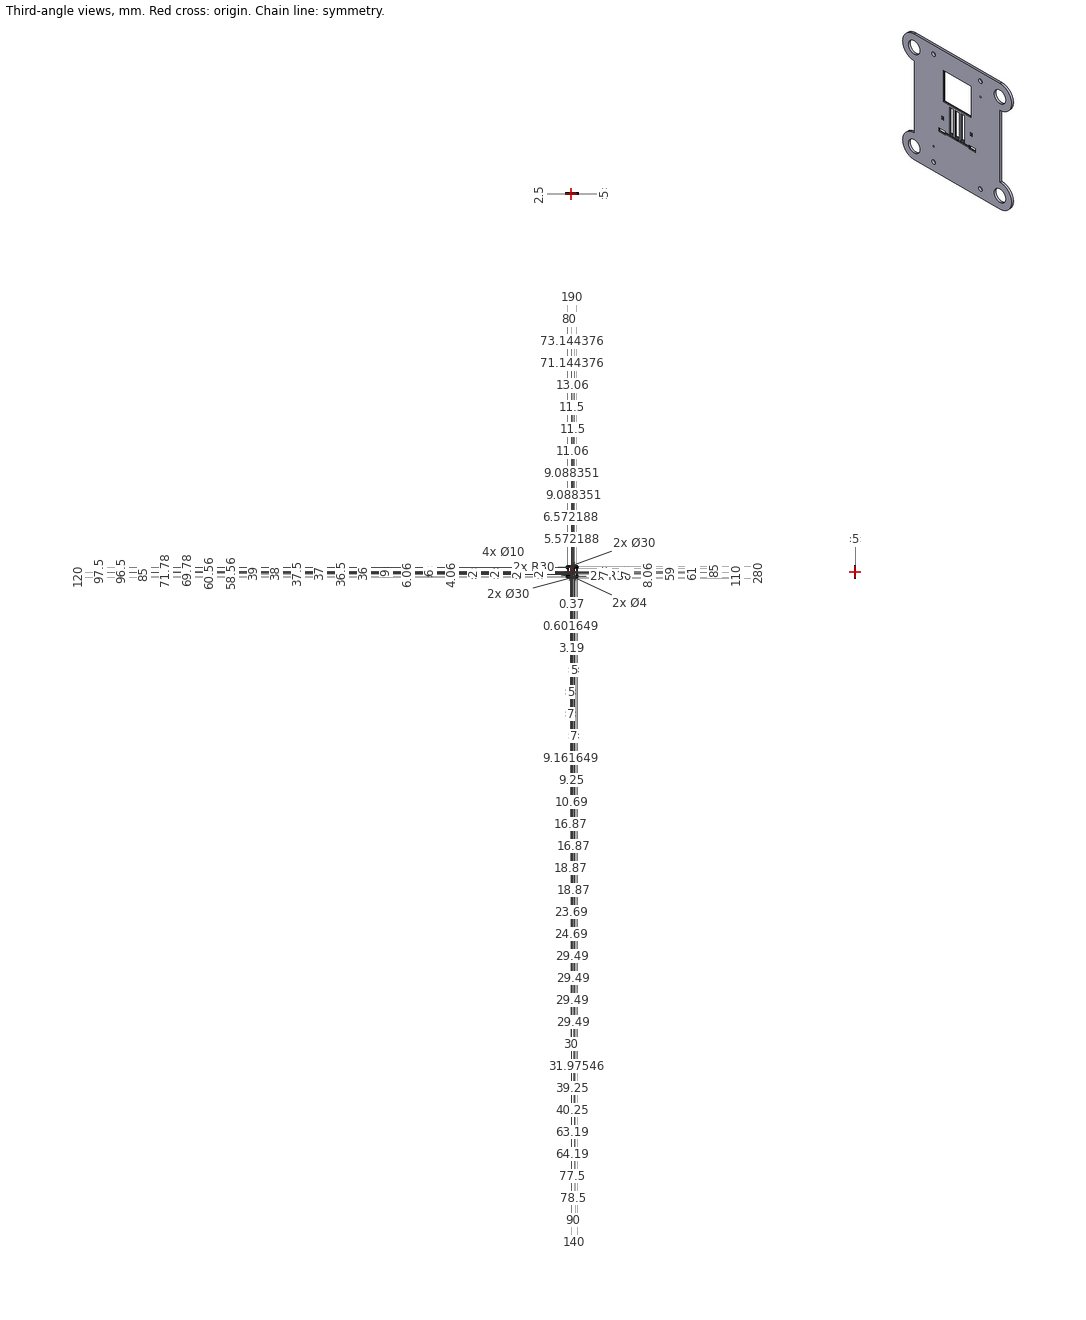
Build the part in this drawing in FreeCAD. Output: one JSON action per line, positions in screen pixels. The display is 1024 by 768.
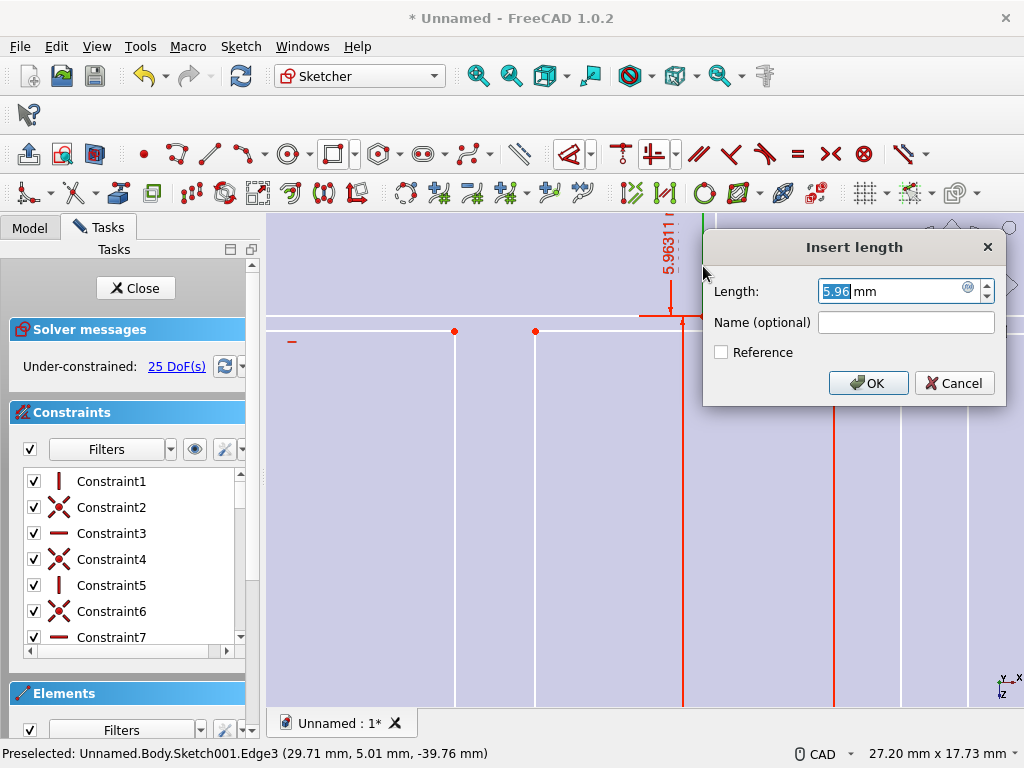
{"action": "type", "text": "6.06"}
{"action": "key", "text": "Return"}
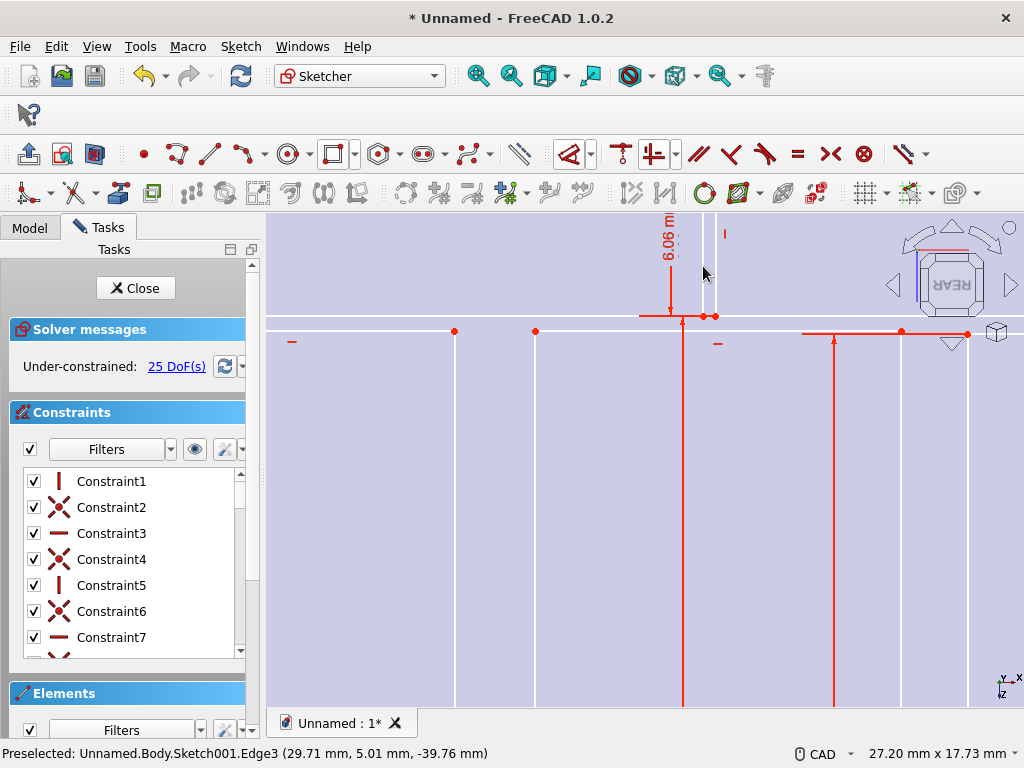
{"action": "scroll", "coordinate": [566, 329], "scroll_direction": "down", "scroll_amount": 13}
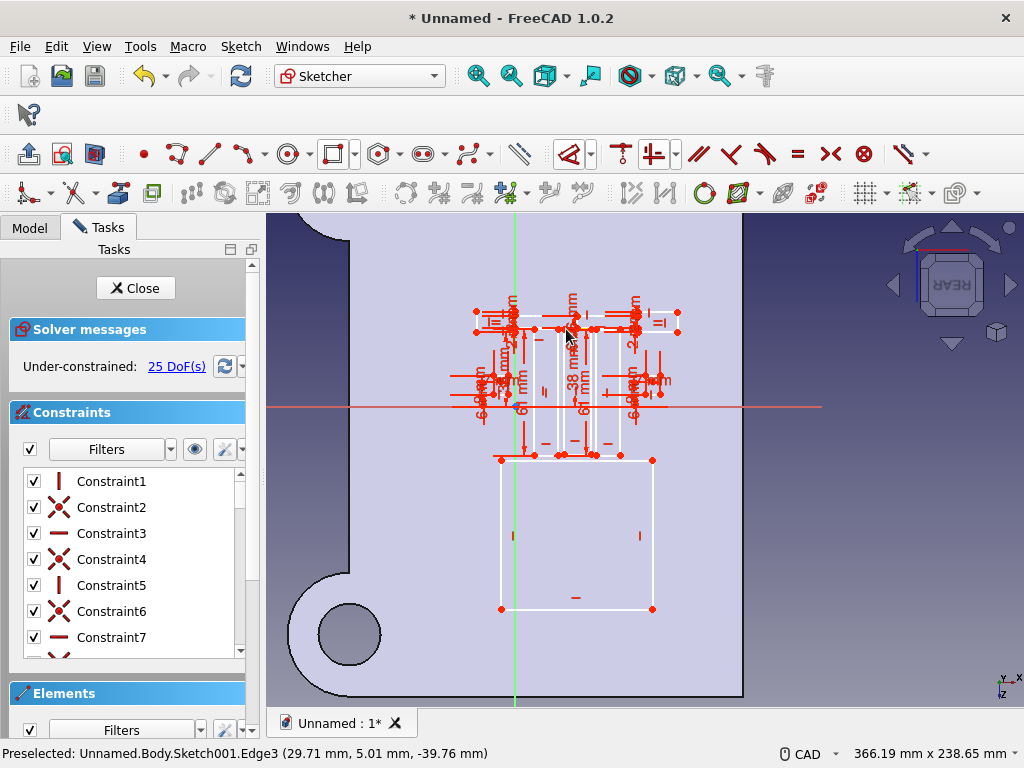
{"action": "scroll", "coordinate": [603, 456], "scroll_direction": "up", "scroll_amount": 6}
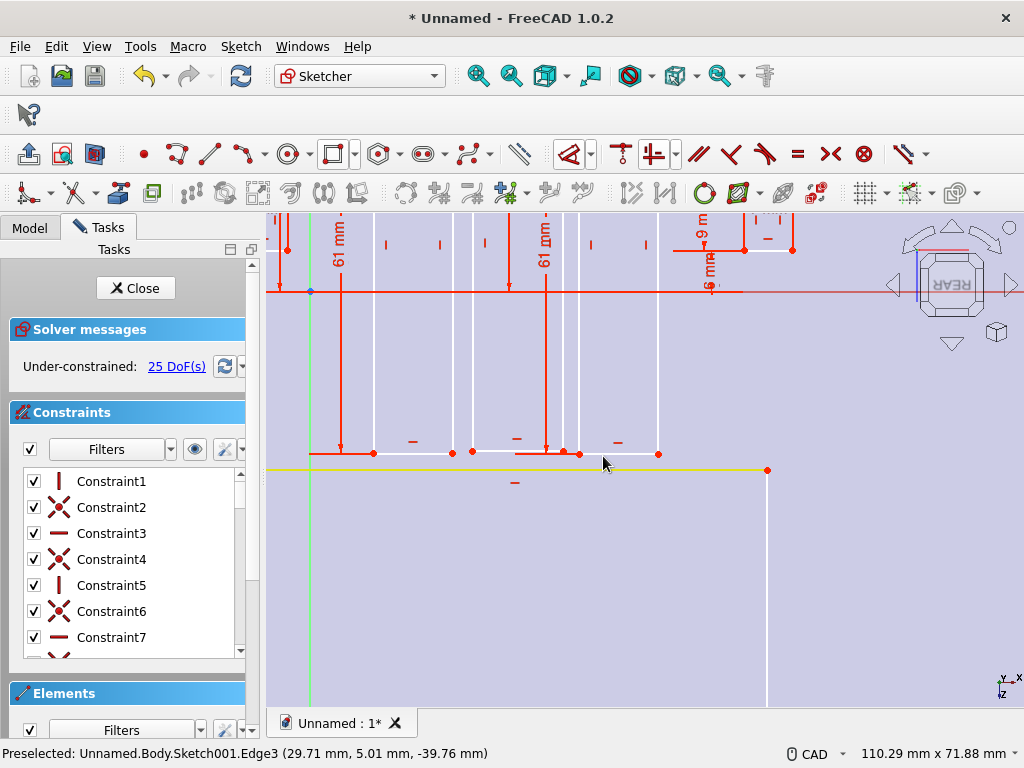
{"action": "left_click", "coordinate": [603, 454]}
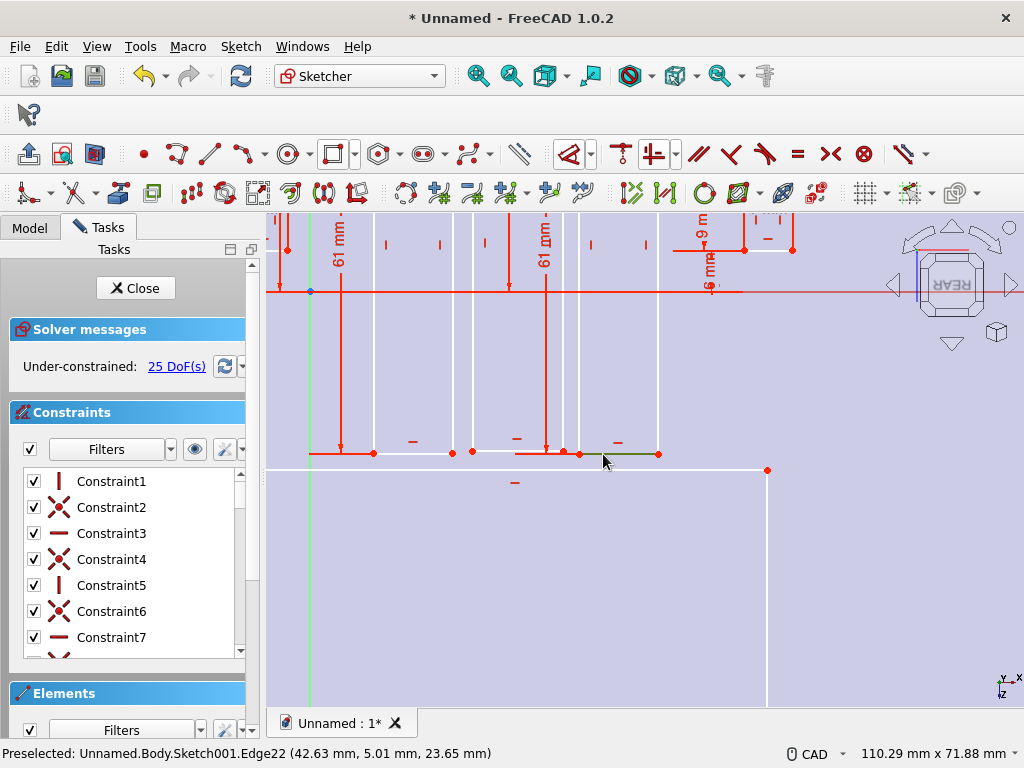
{"action": "key", "text": "l"}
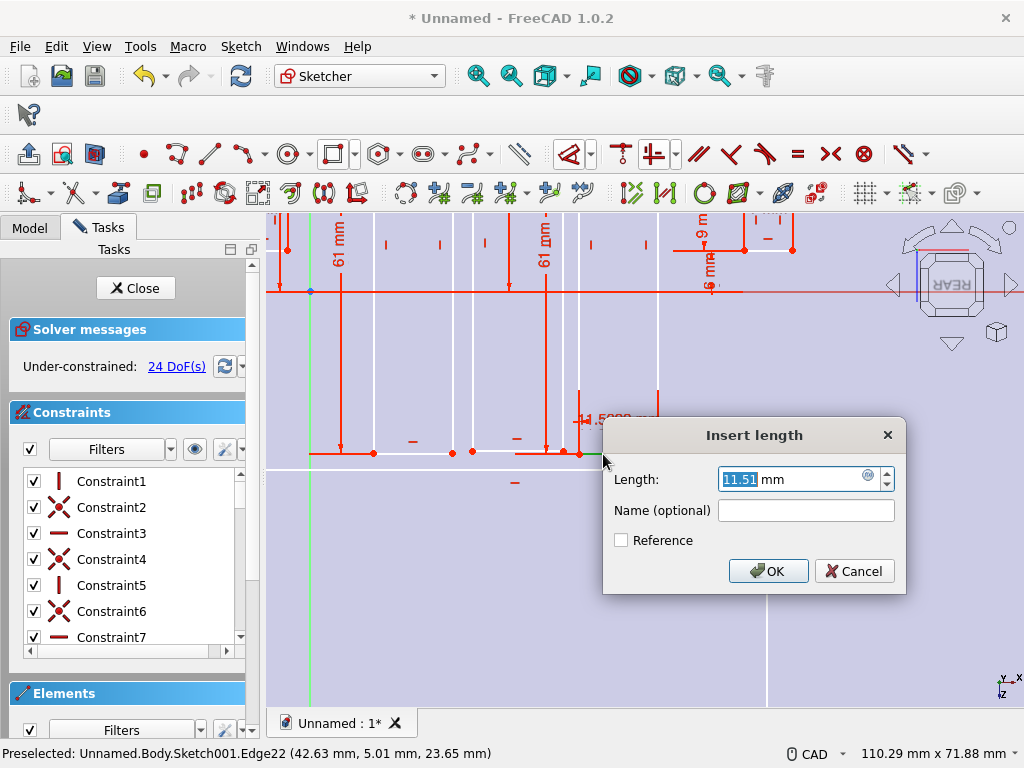
{"action": "type", "text": "11.5"}
{"action": "key", "text": "Return"}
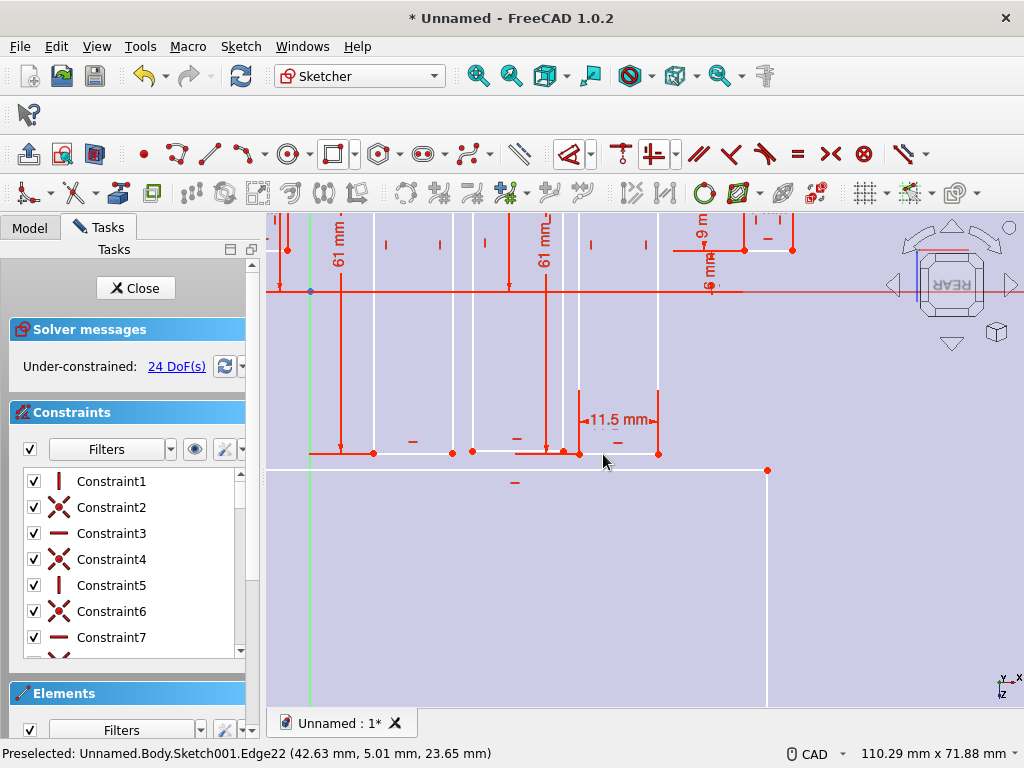
{"action": "left_click", "coordinate": [397, 454]}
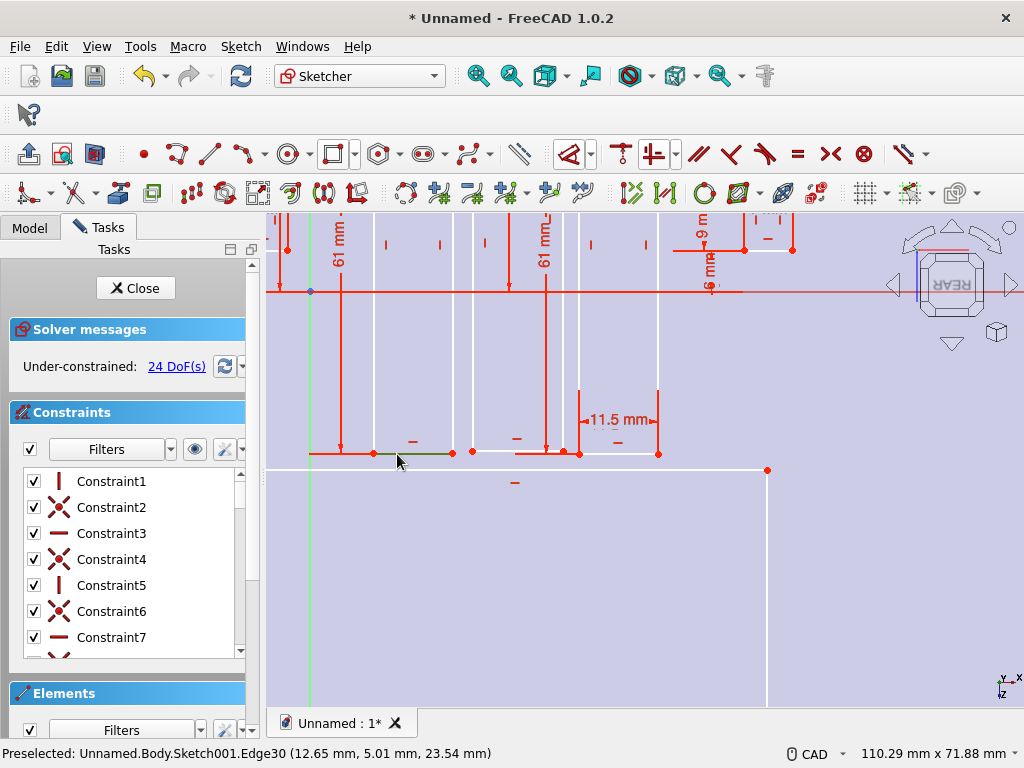
{"action": "key", "text": "l"}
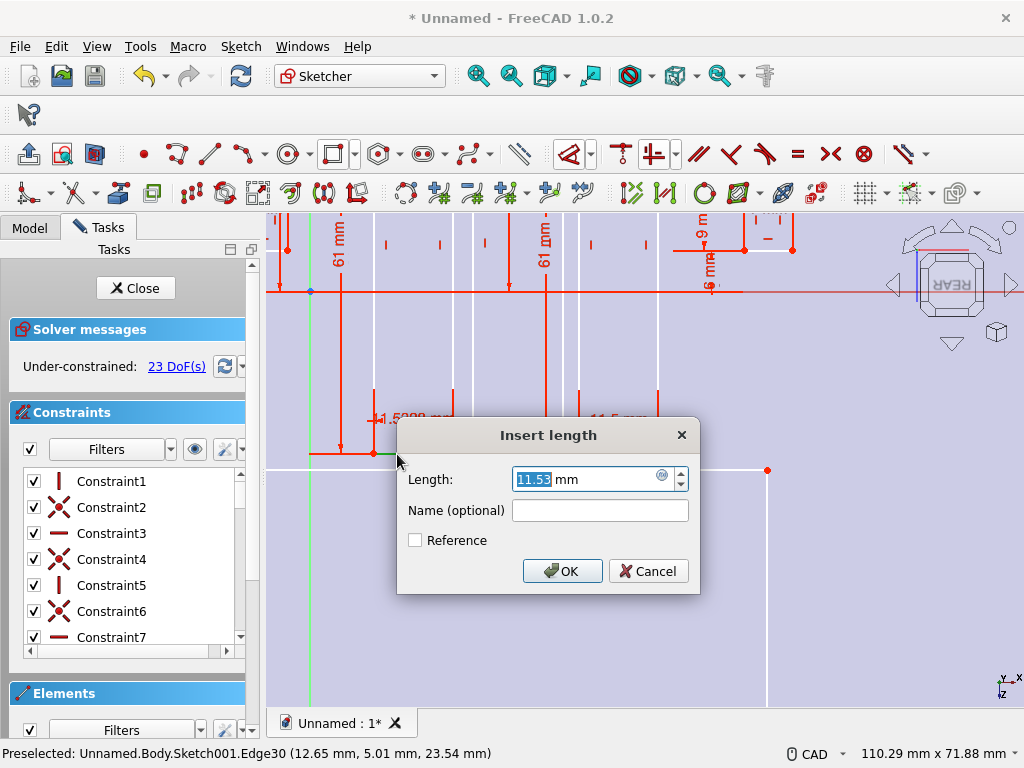
{"action": "type", "text": "11.5"}
{"action": "key", "text": "Return"}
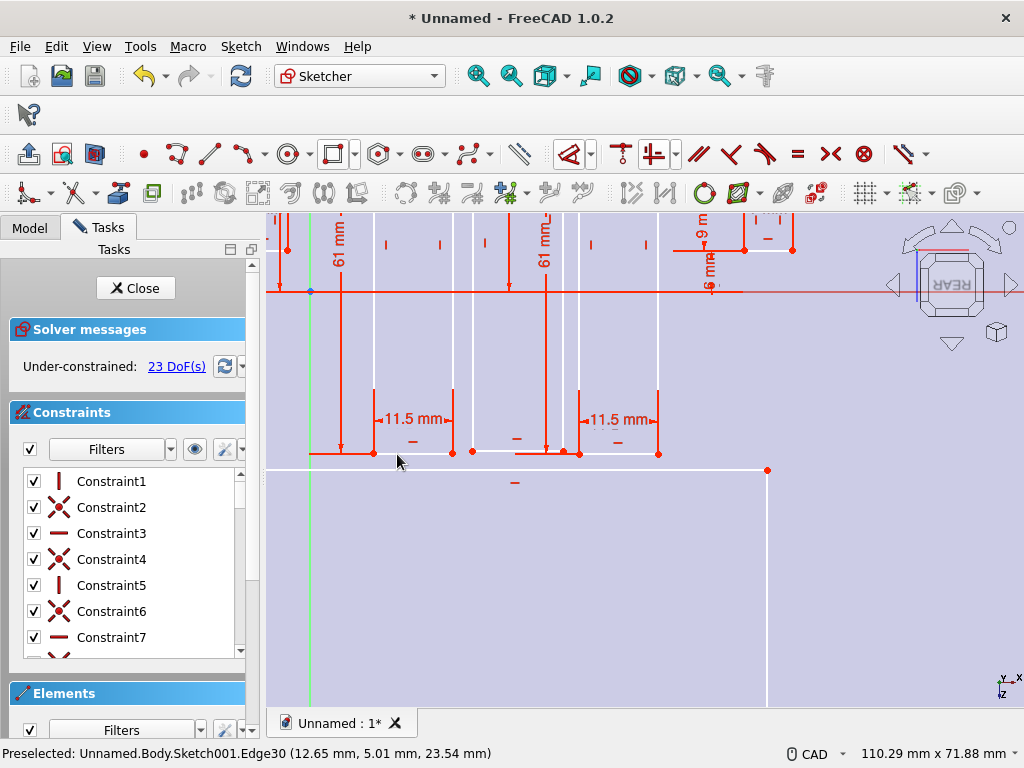
{"action": "scroll", "coordinate": [602, 456], "scroll_direction": "down", "scroll_amount": 6}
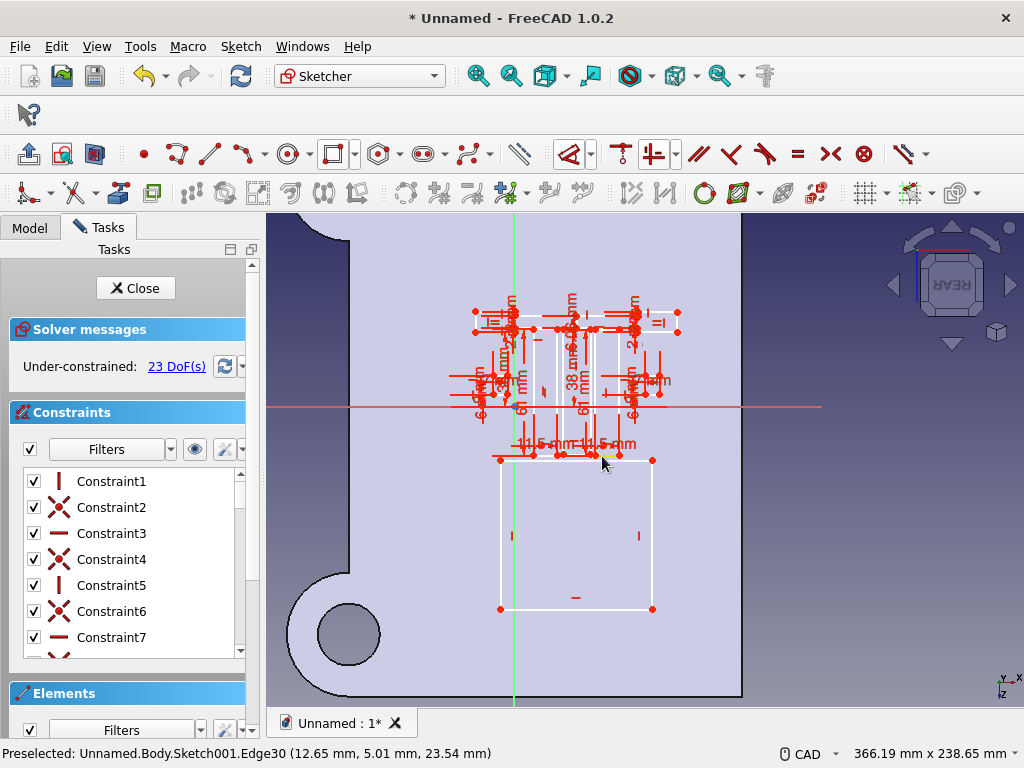
{"action": "scroll", "coordinate": [577, 320], "scroll_direction": "up", "scroll_amount": 14}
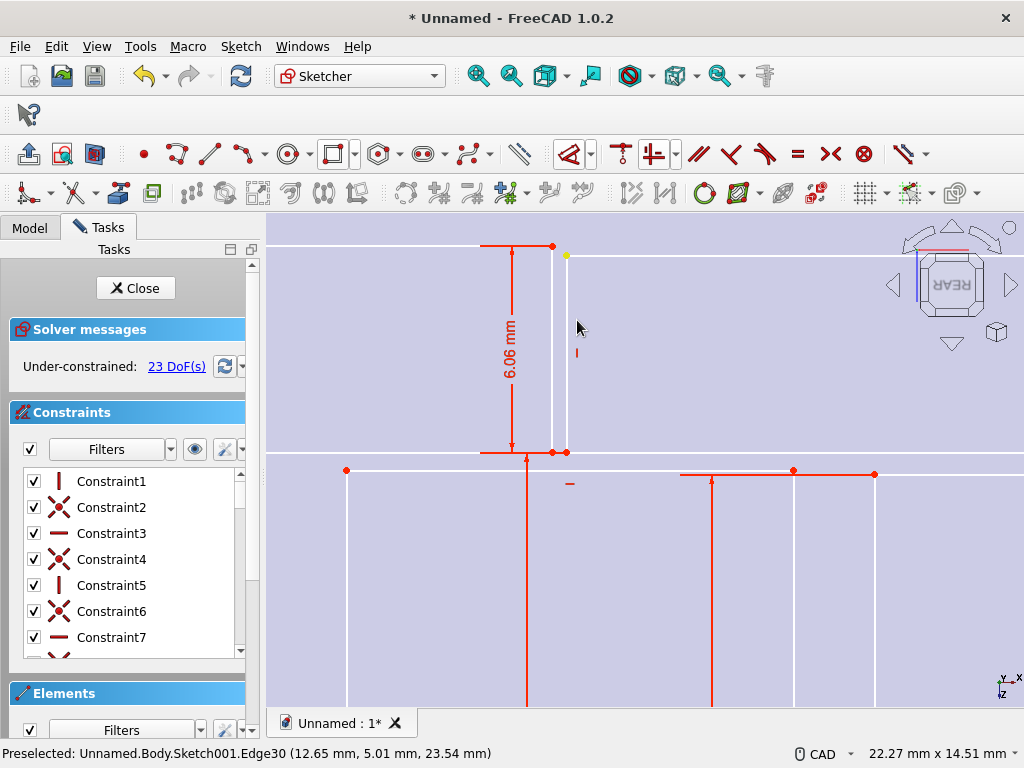
{"action": "left_click", "coordinate": [567, 315]}